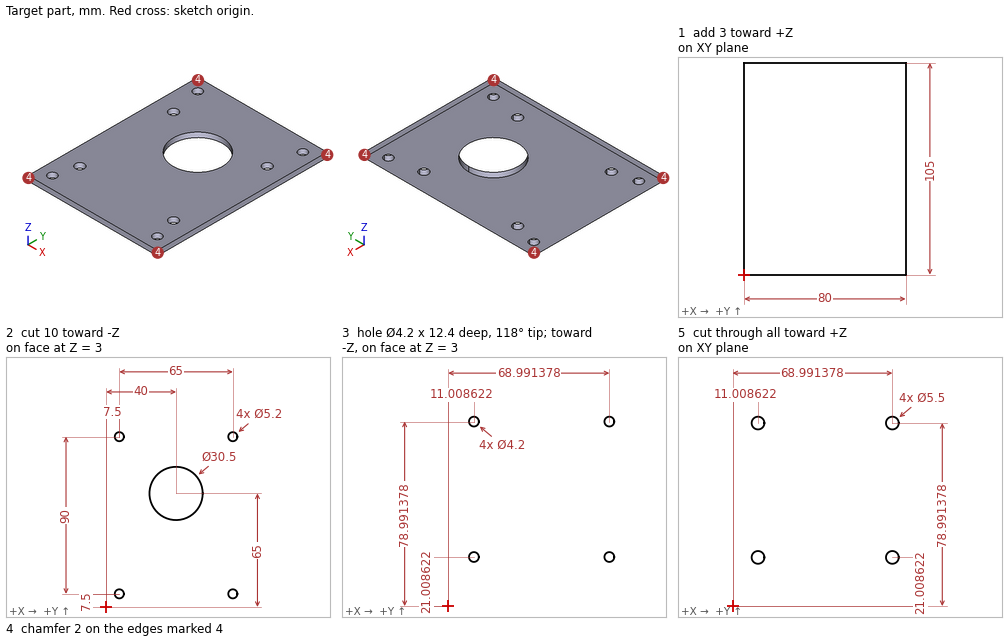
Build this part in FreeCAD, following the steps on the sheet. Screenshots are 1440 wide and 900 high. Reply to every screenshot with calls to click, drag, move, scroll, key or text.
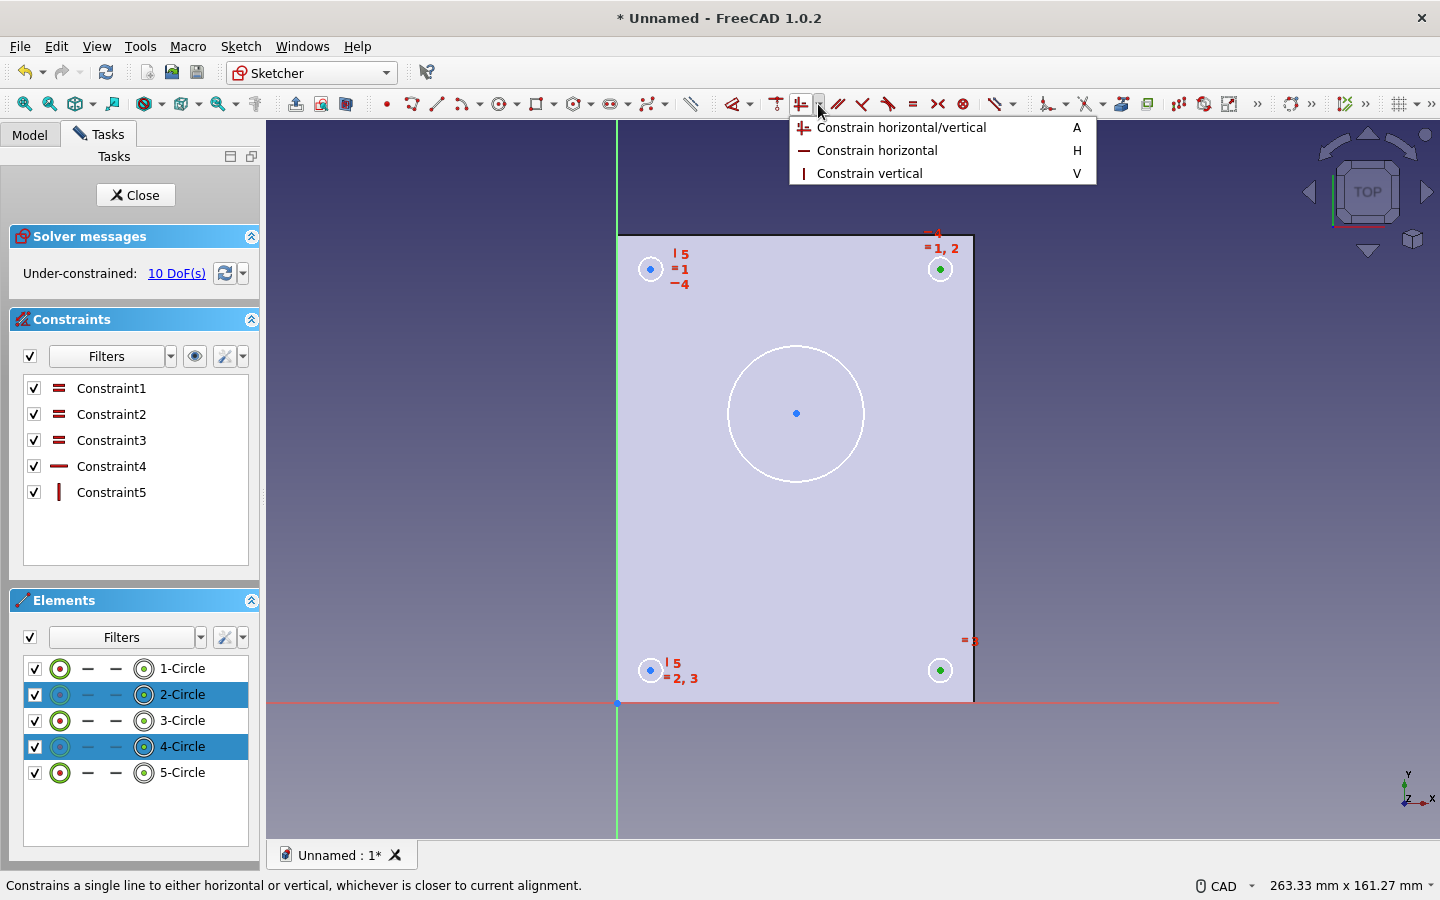
click(943, 174)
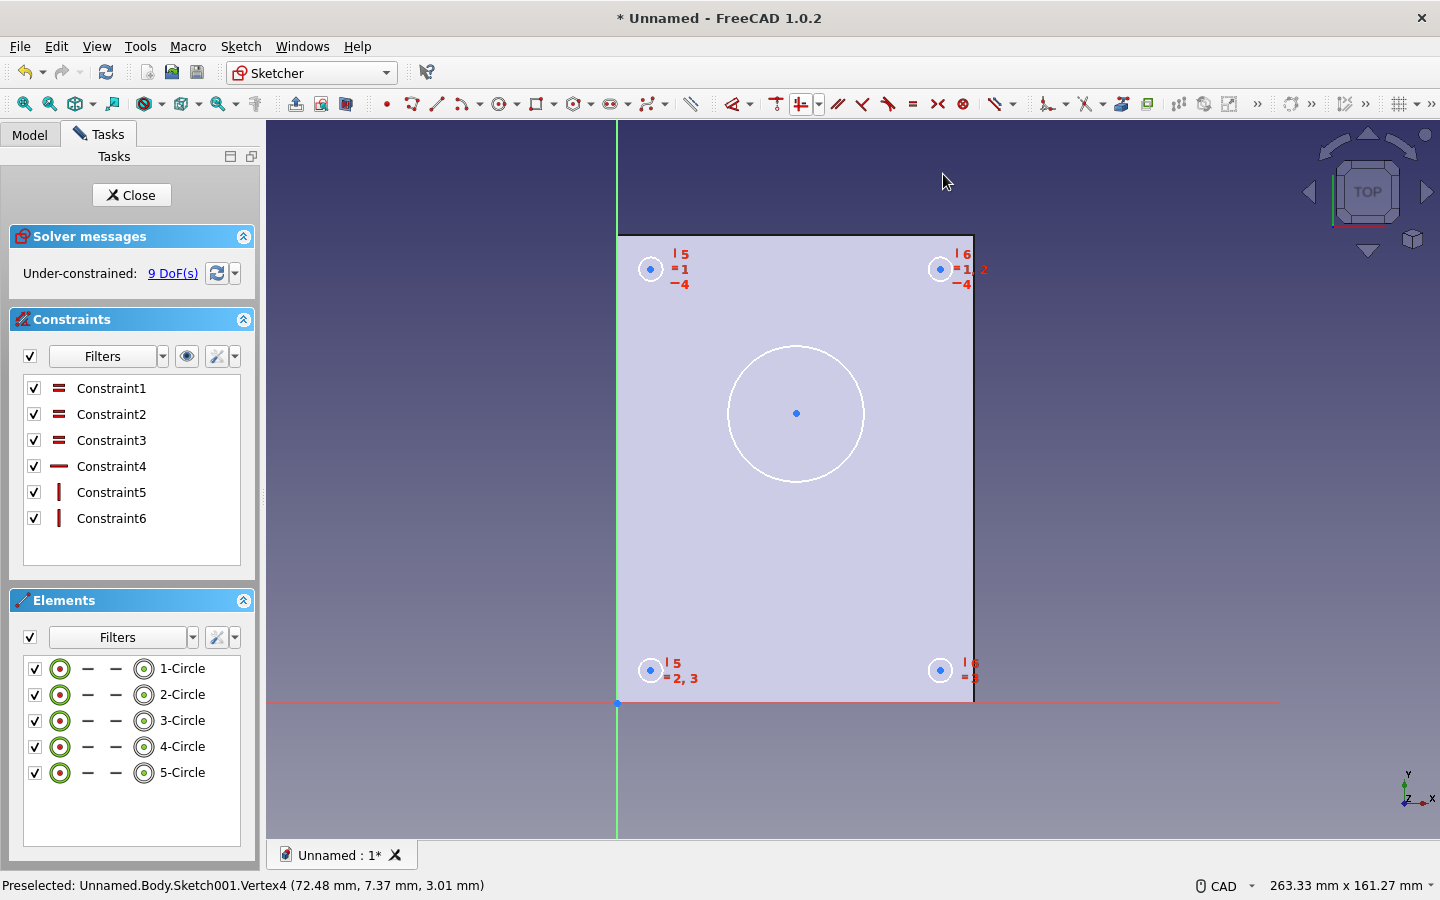
click(651, 670)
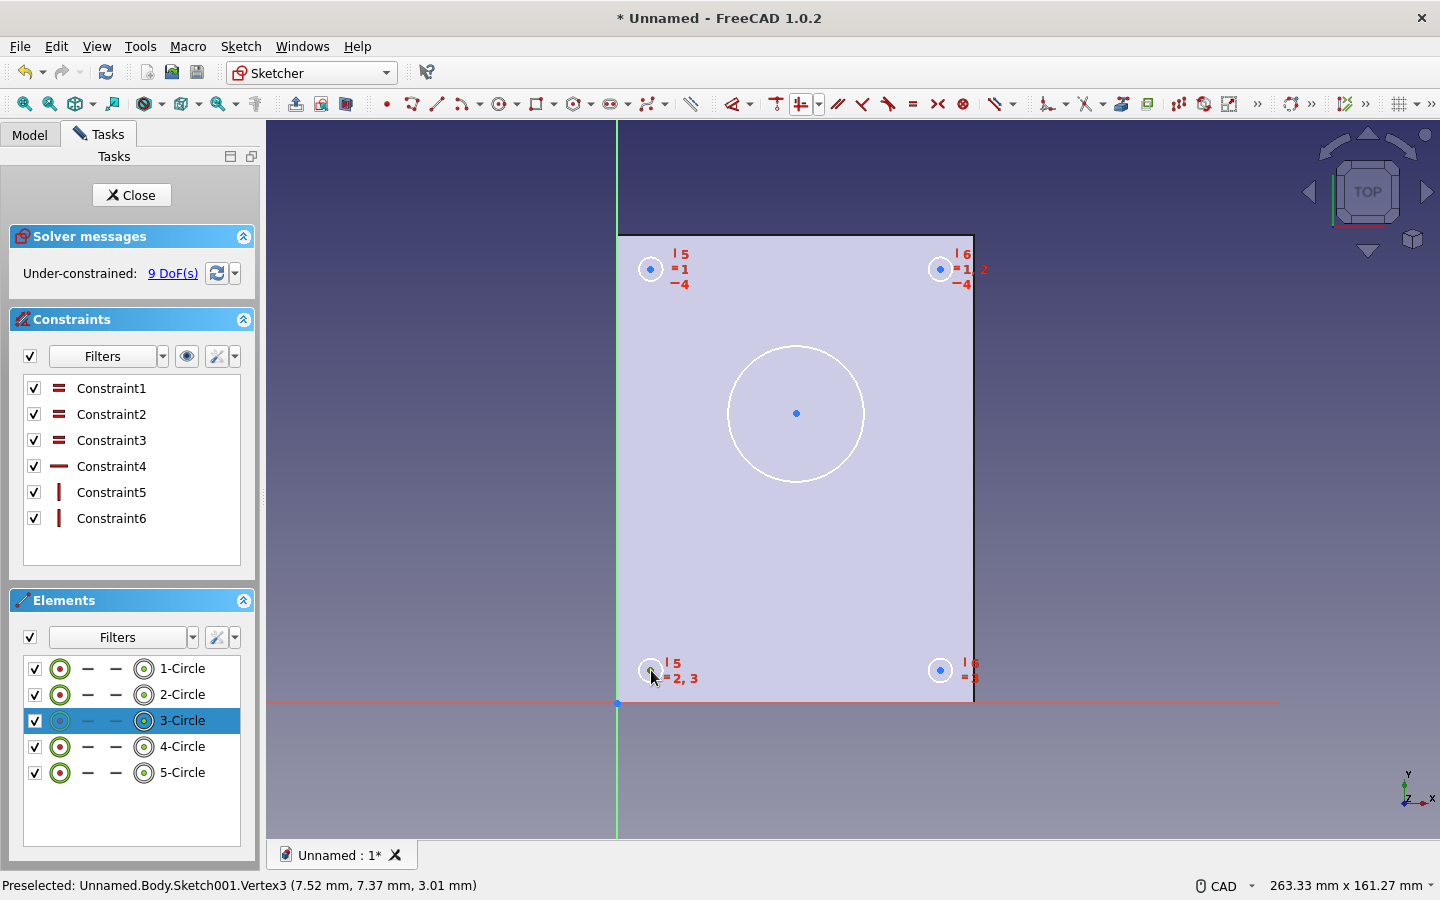
click(940, 670)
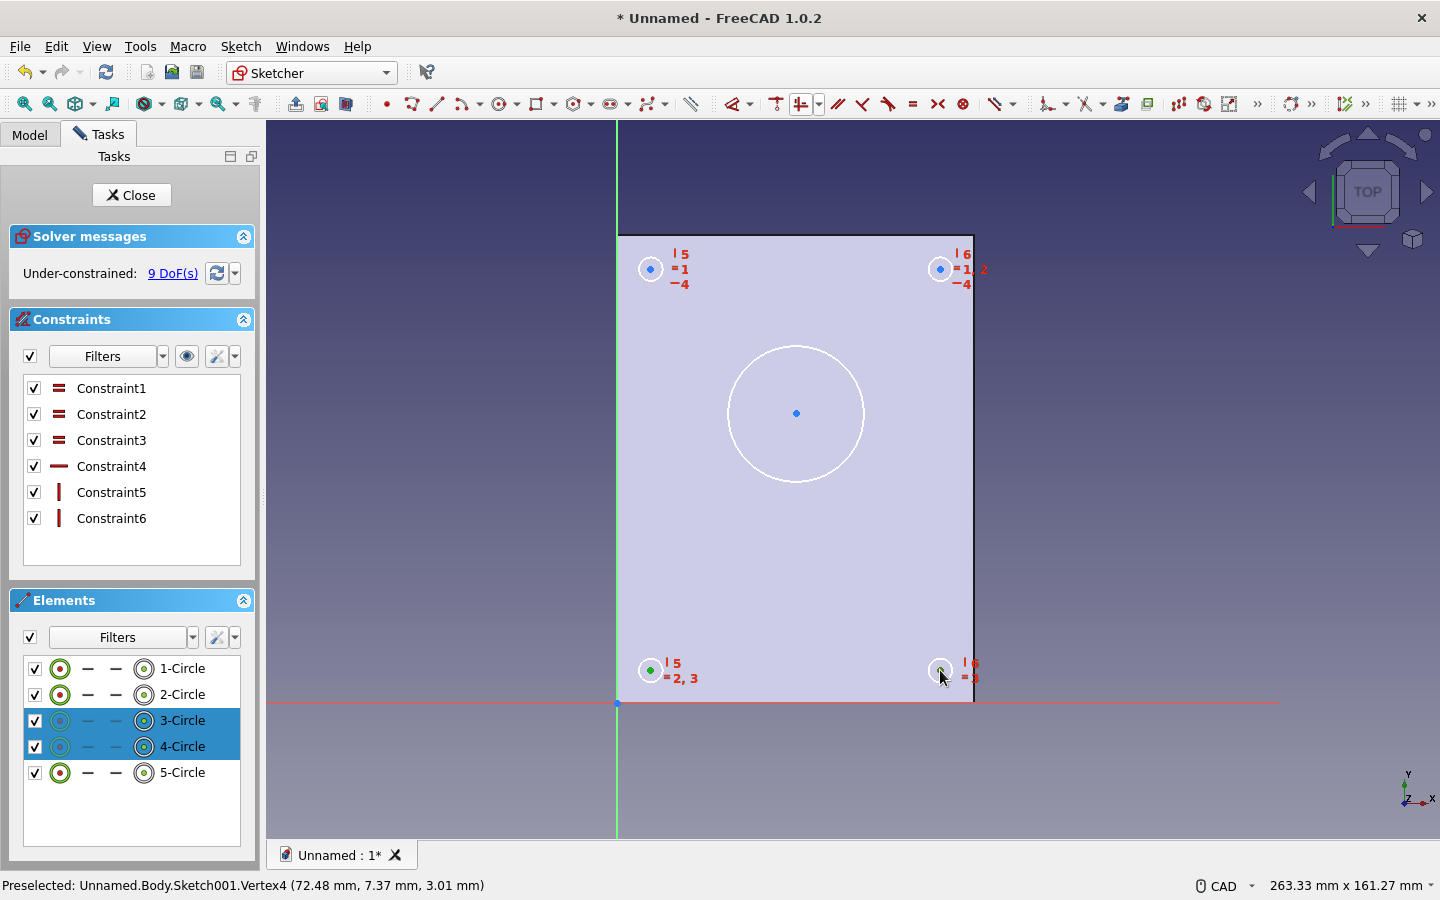
click(818, 104)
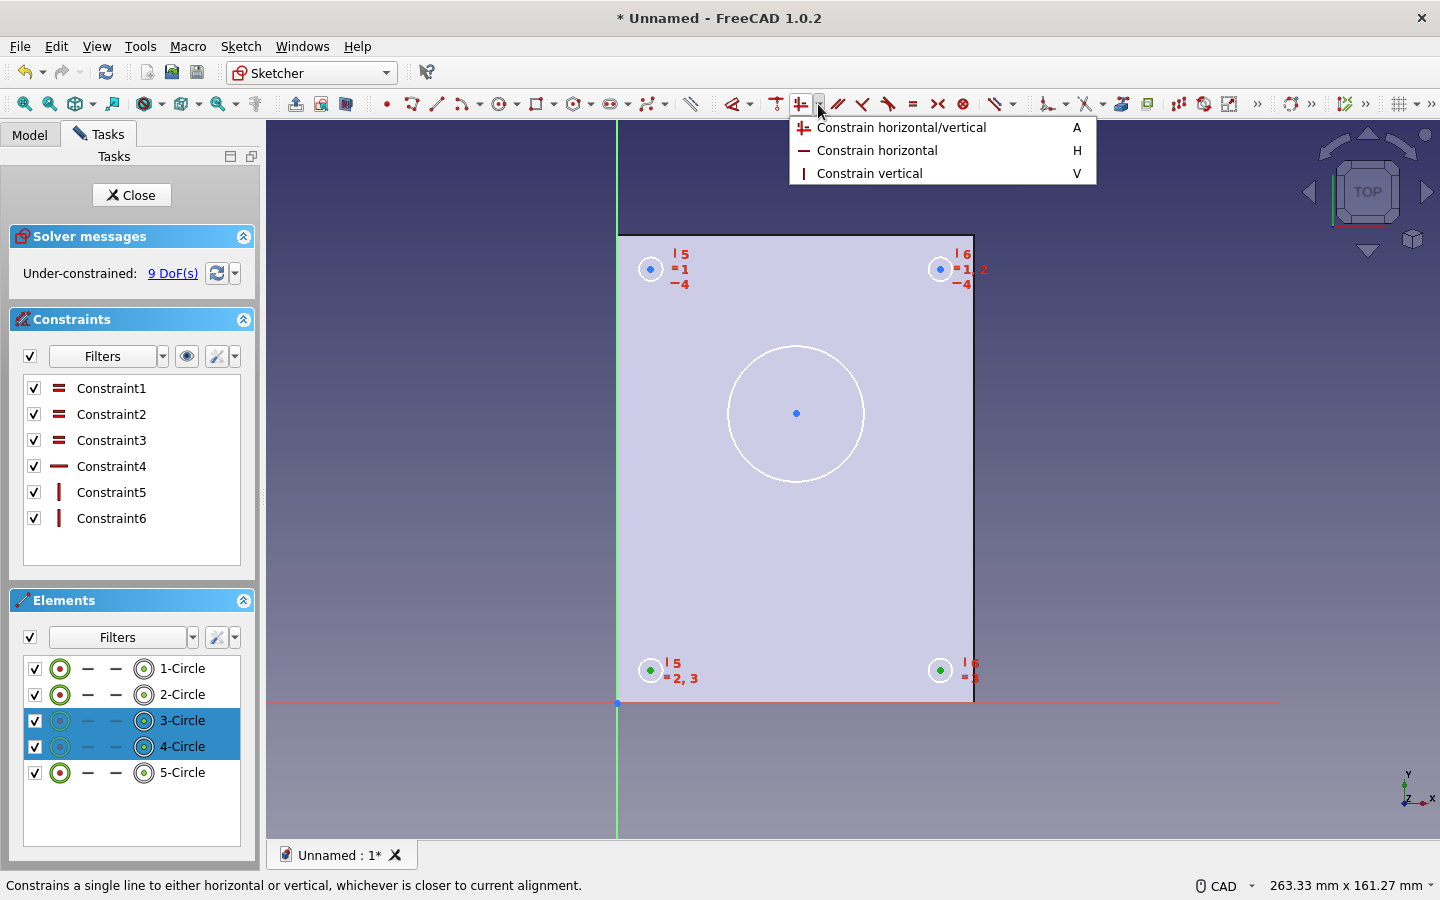
click(943, 150)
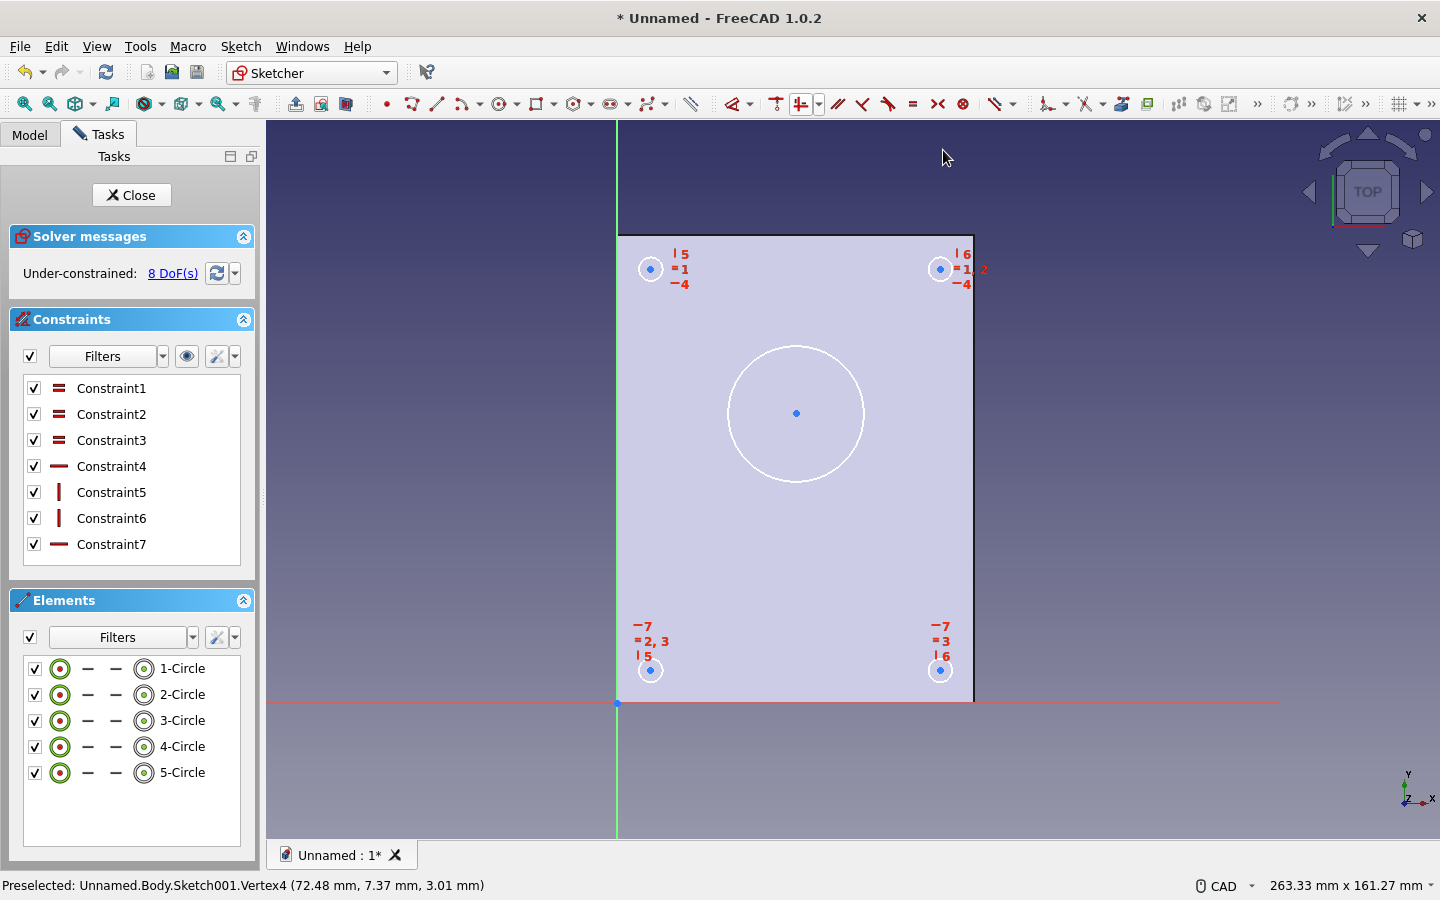
click(732, 104)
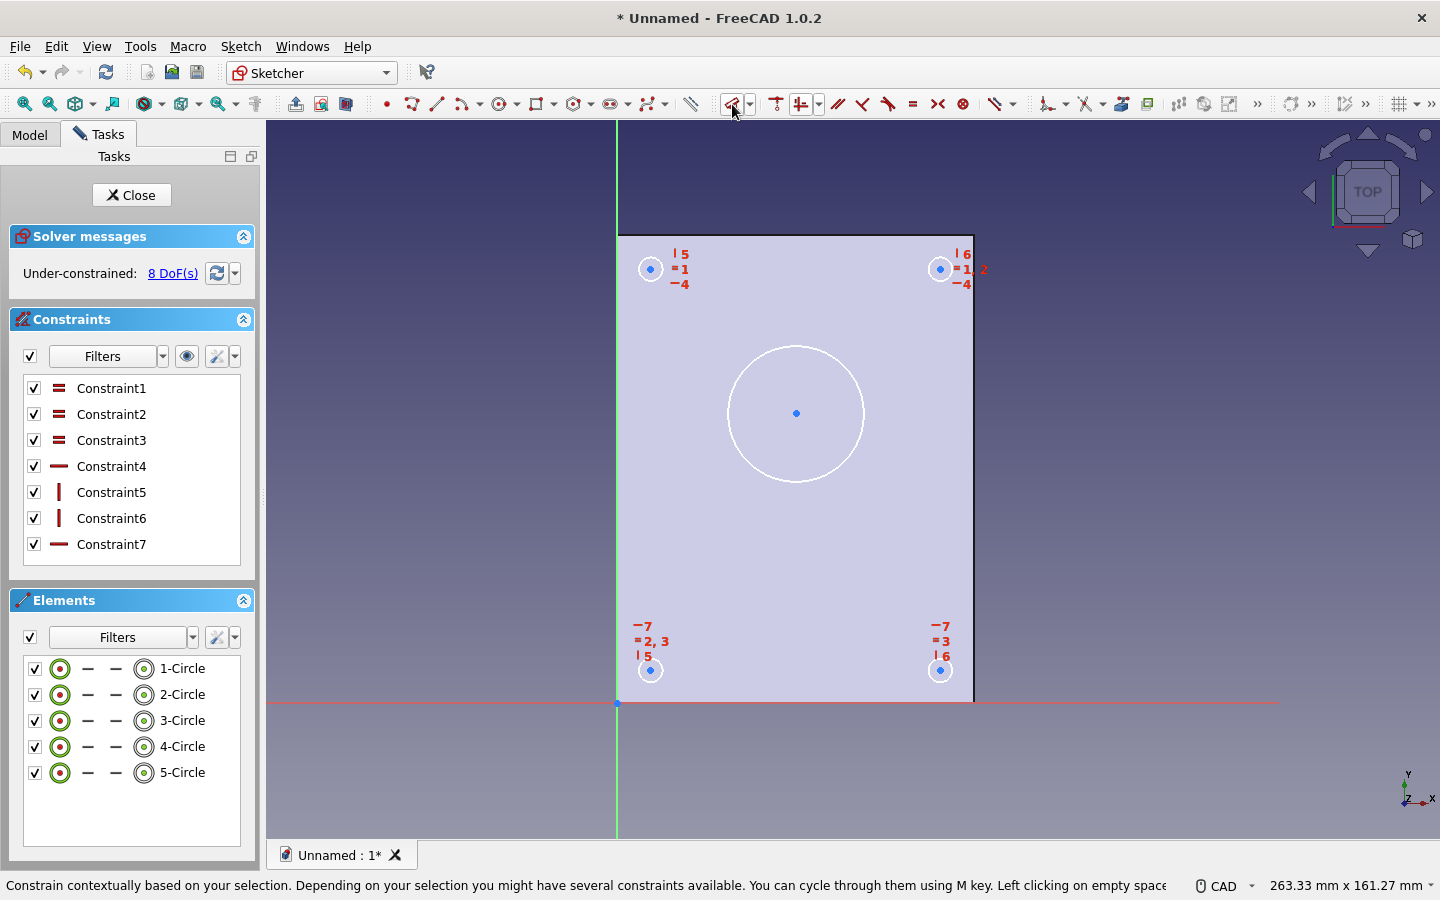
scroll(659, 261, up, 3)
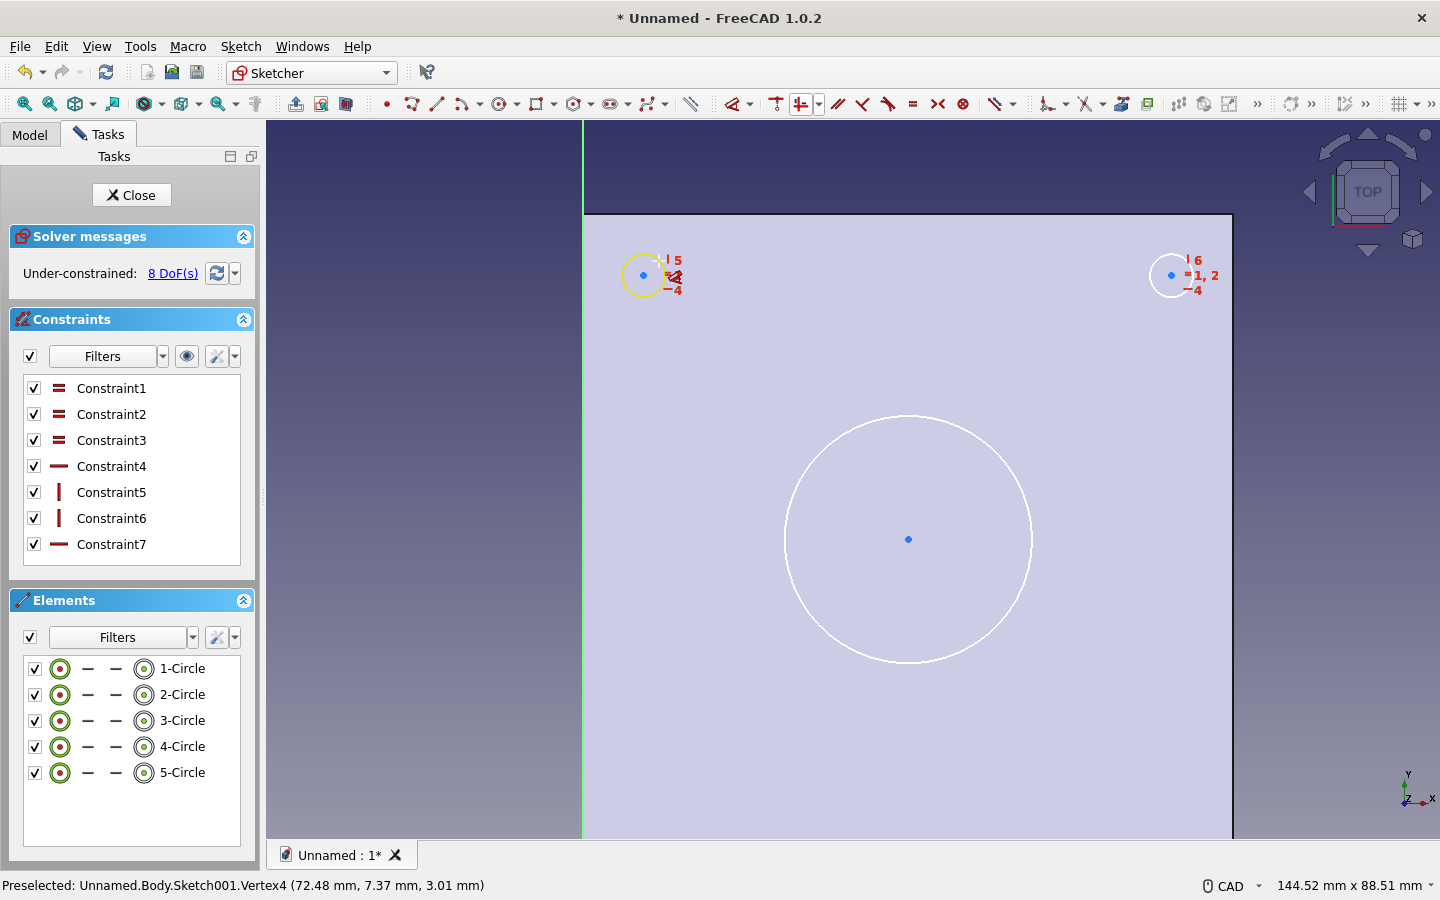
click(659, 261)
click(682, 239)